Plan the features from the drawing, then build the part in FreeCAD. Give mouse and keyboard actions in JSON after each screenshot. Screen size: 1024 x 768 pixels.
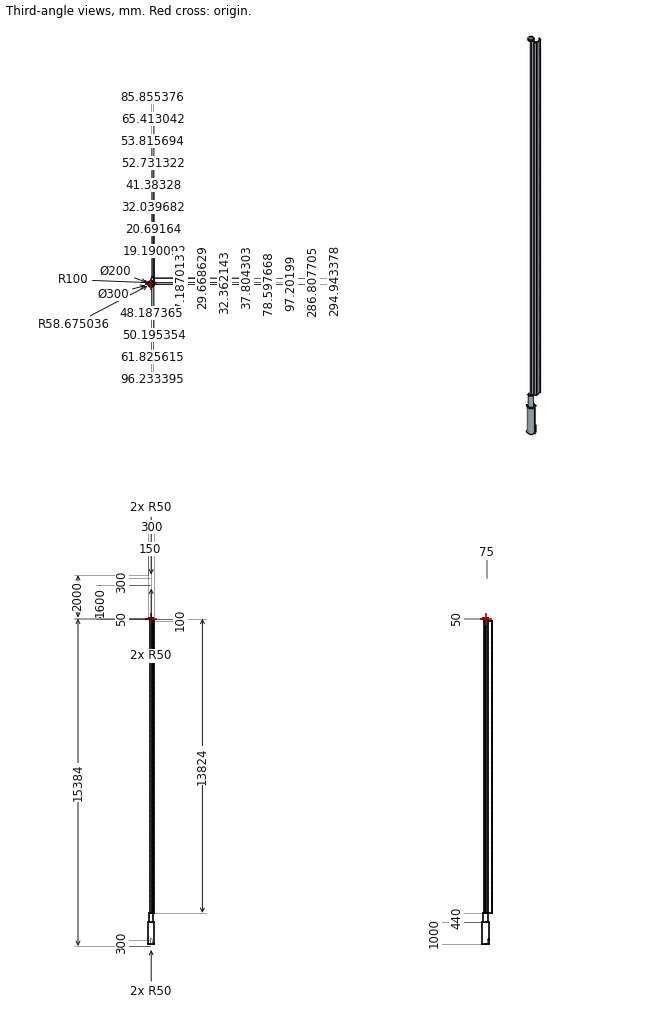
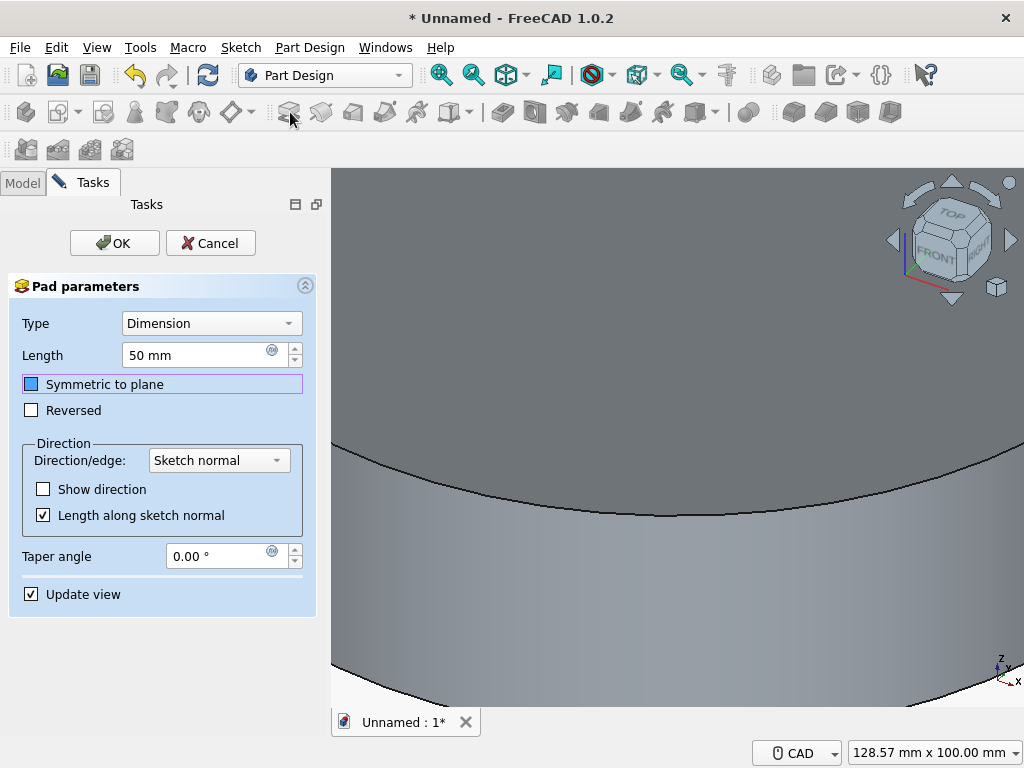
{"action": "left_click", "coordinate": [115, 243]}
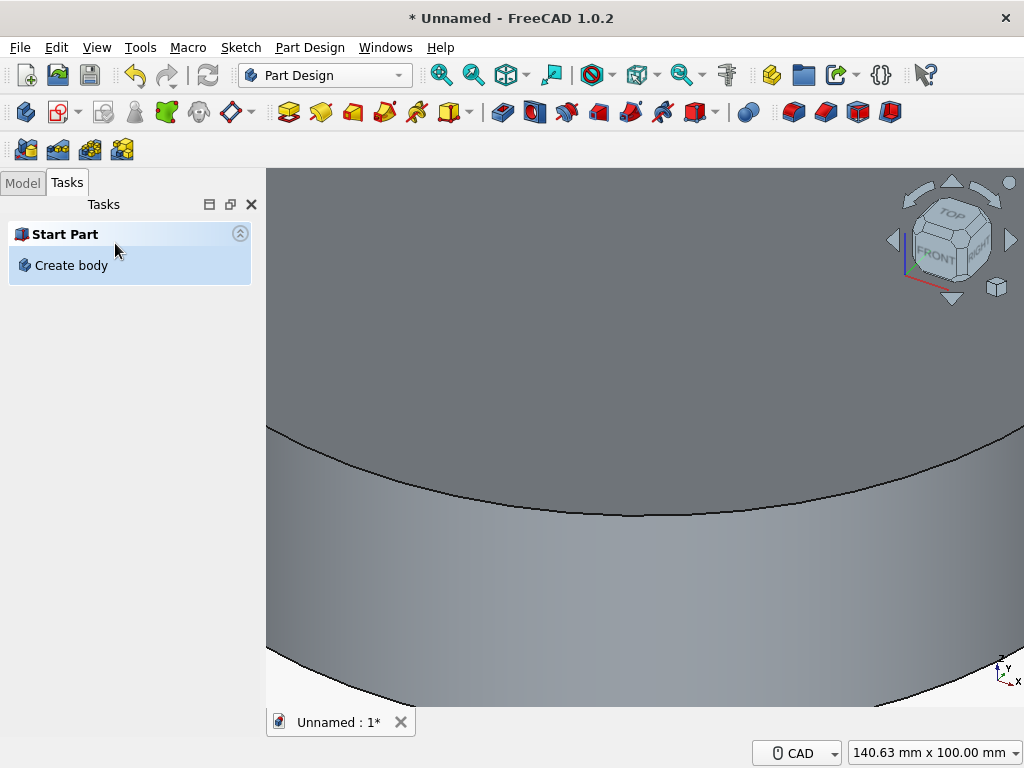
{"action": "left_click", "coordinate": [442, 76]}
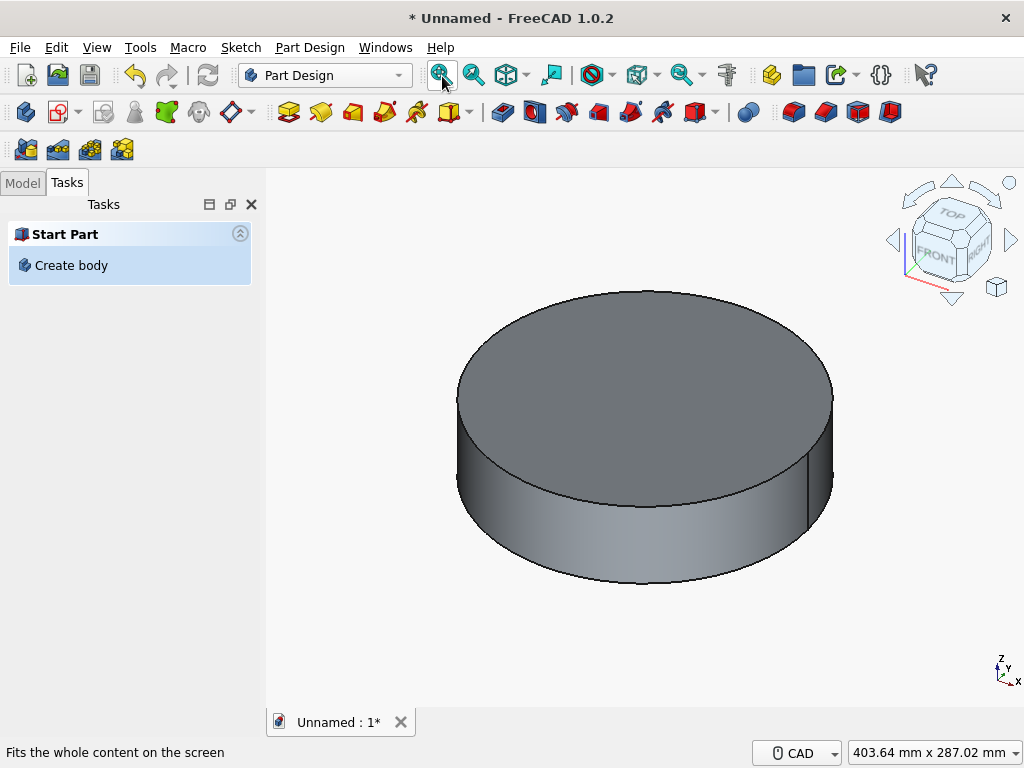
{"action": "left_click", "coordinate": [58, 112]}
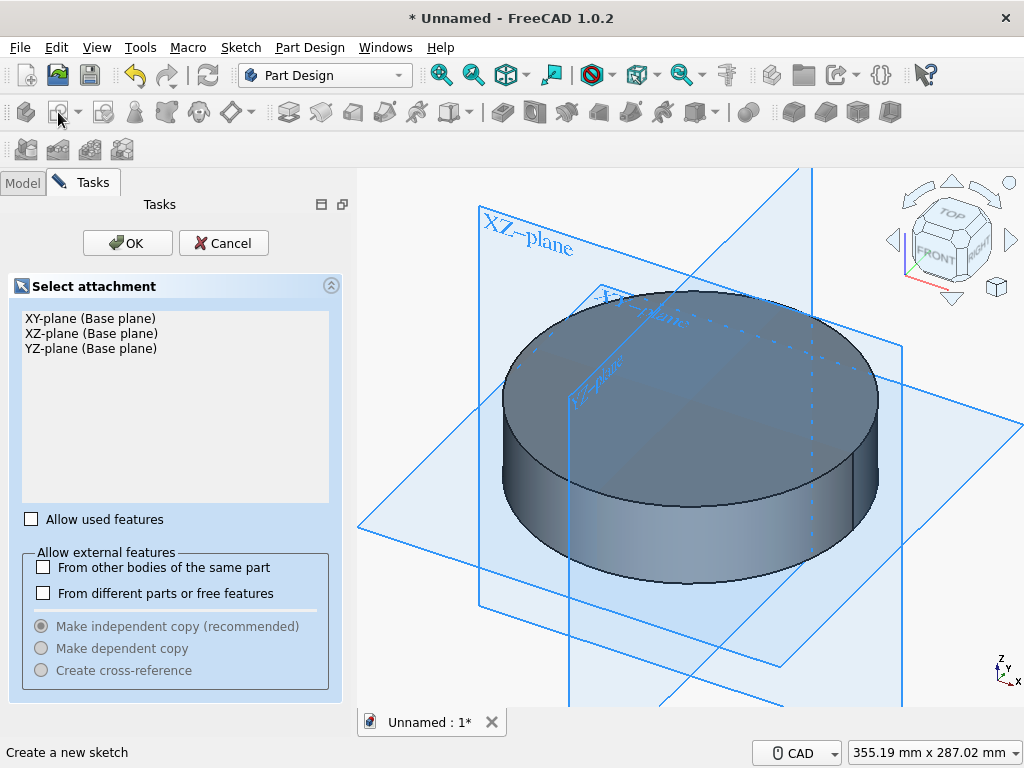
{"action": "left_click", "coordinate": [82, 318]}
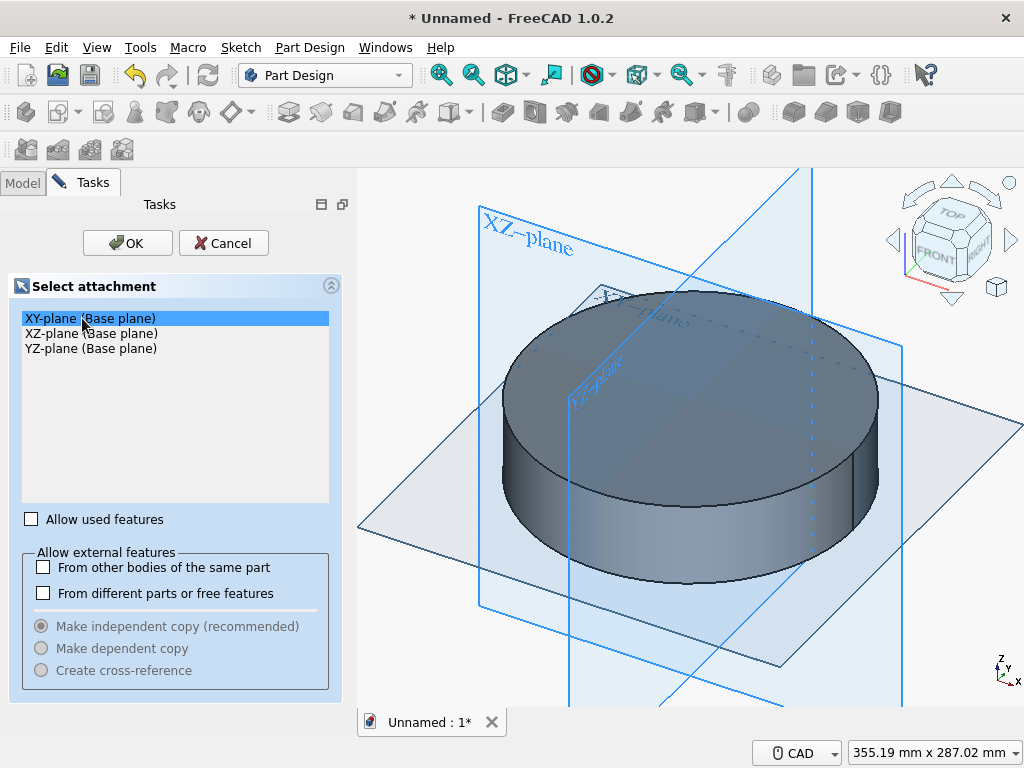
{"action": "left_click", "coordinate": [128, 243]}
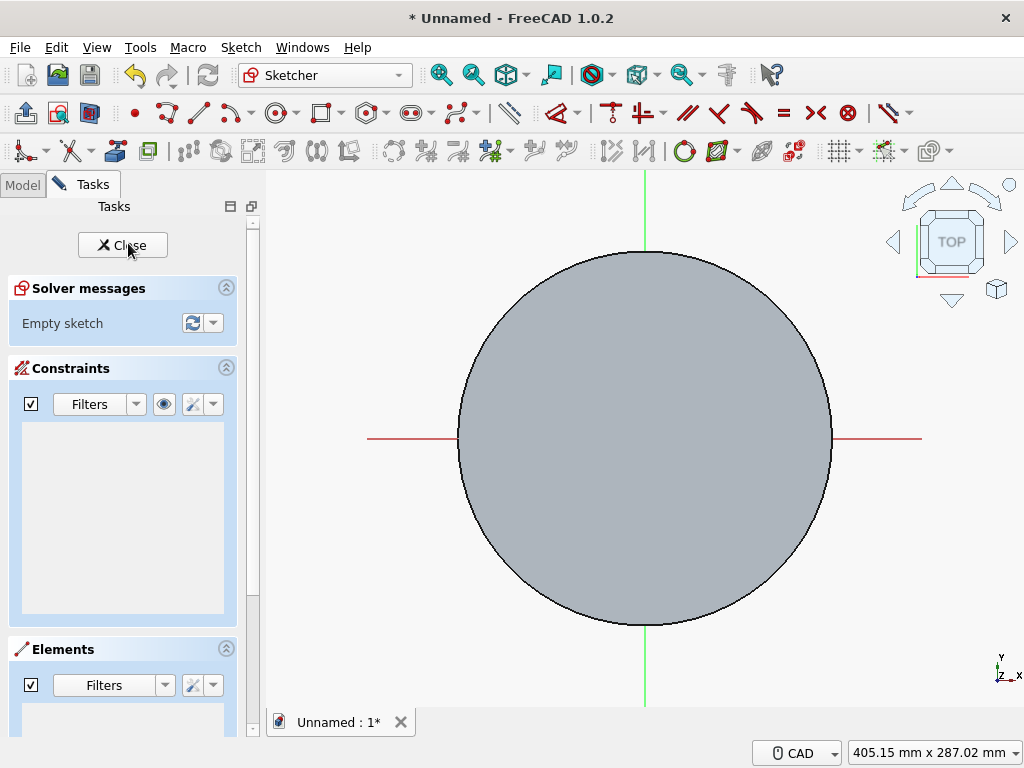
{"action": "left_click", "coordinate": [90, 114]}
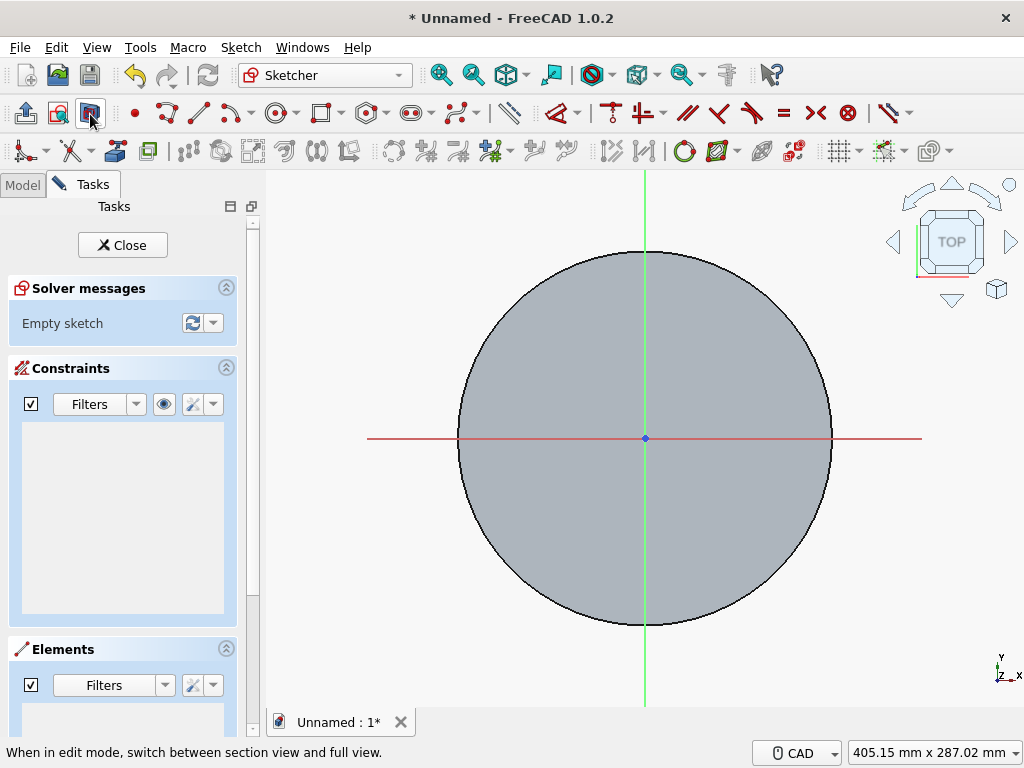
{"action": "scroll", "coordinate": [449, 661], "scroll_direction": "down", "scroll_amount": 4}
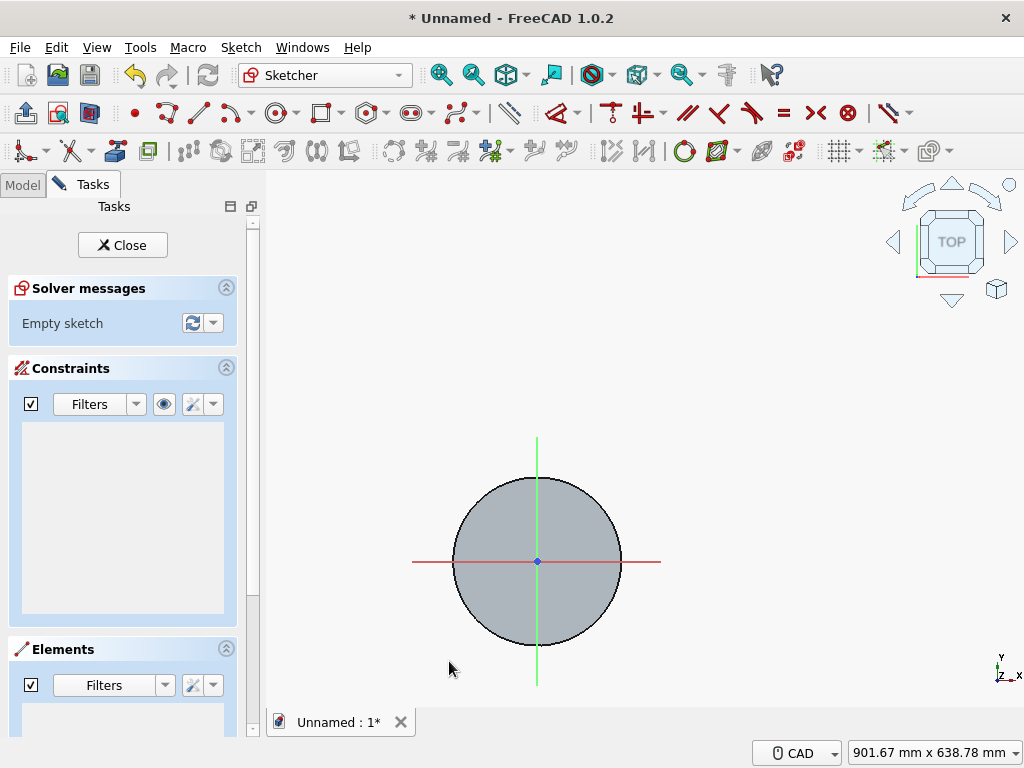
{"action": "left_click", "coordinate": [168, 114]}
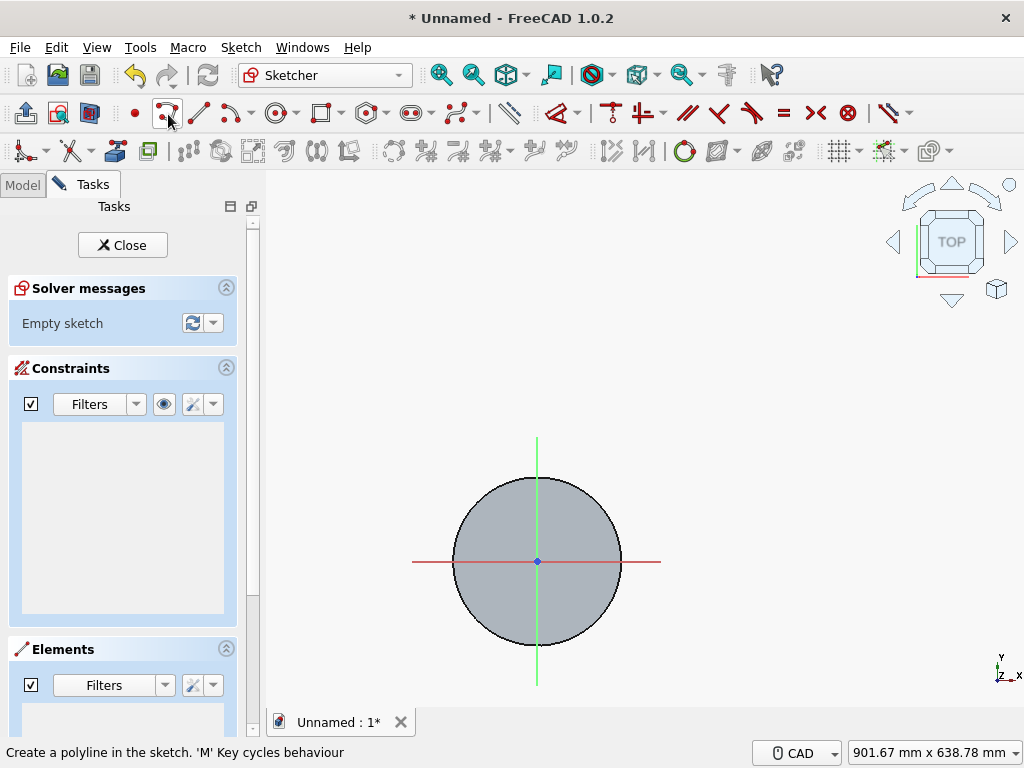
{"action": "left_click", "coordinate": [537, 512]}
{"action": "left_click", "coordinate": [589, 495]}
{"action": "left_click", "coordinate": [644, 468]}
{"action": "left_click", "coordinate": [627, 320]}
{"action": "left_click", "coordinate": [582, 289]}
{"action": "left_click", "coordinate": [609, 289]}
{"action": "left_click", "coordinate": [644, 314]}
{"action": "left_click", "coordinate": [660, 480]}
{"action": "left_click", "coordinate": [618, 539]}
{"action": "left_click", "coordinate": [578, 590]}
{"action": "right_click", "coordinate": [578, 590]}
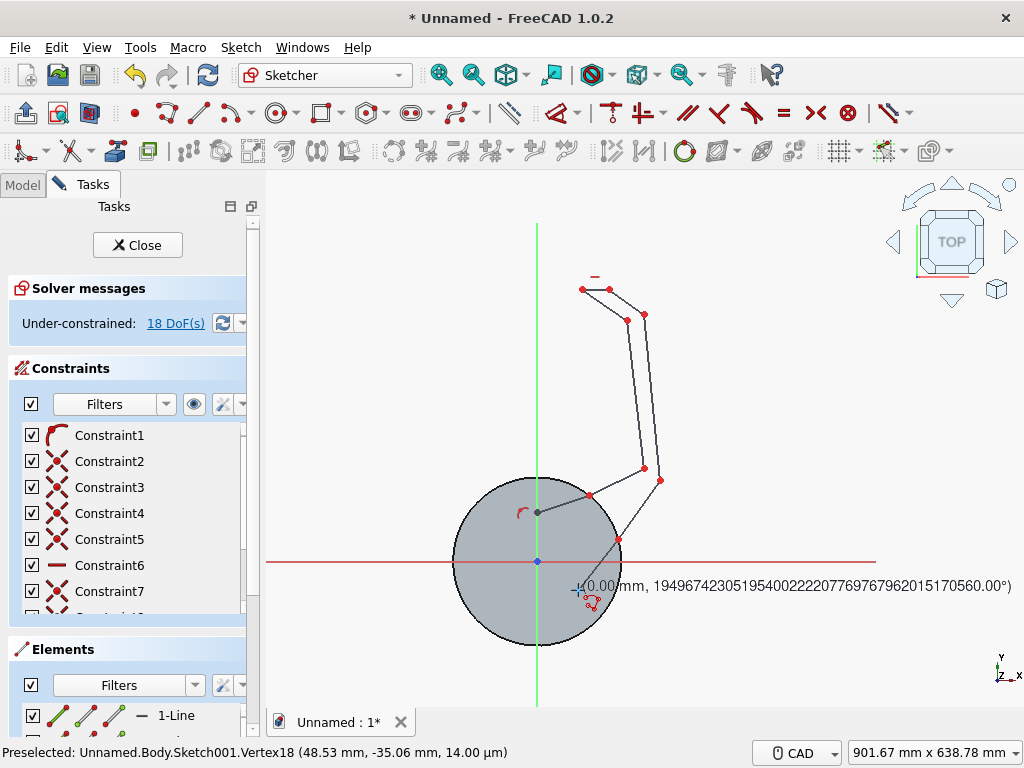
{"action": "left_click", "coordinate": [254, 114]}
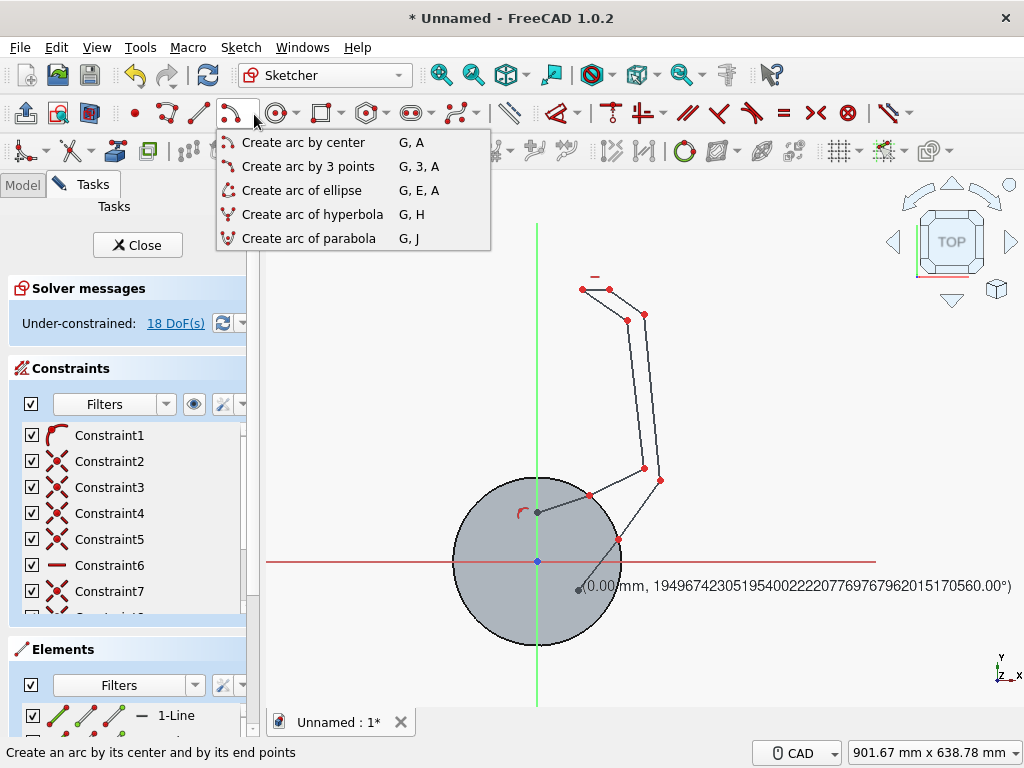
{"action": "left_click", "coordinate": [354, 166]}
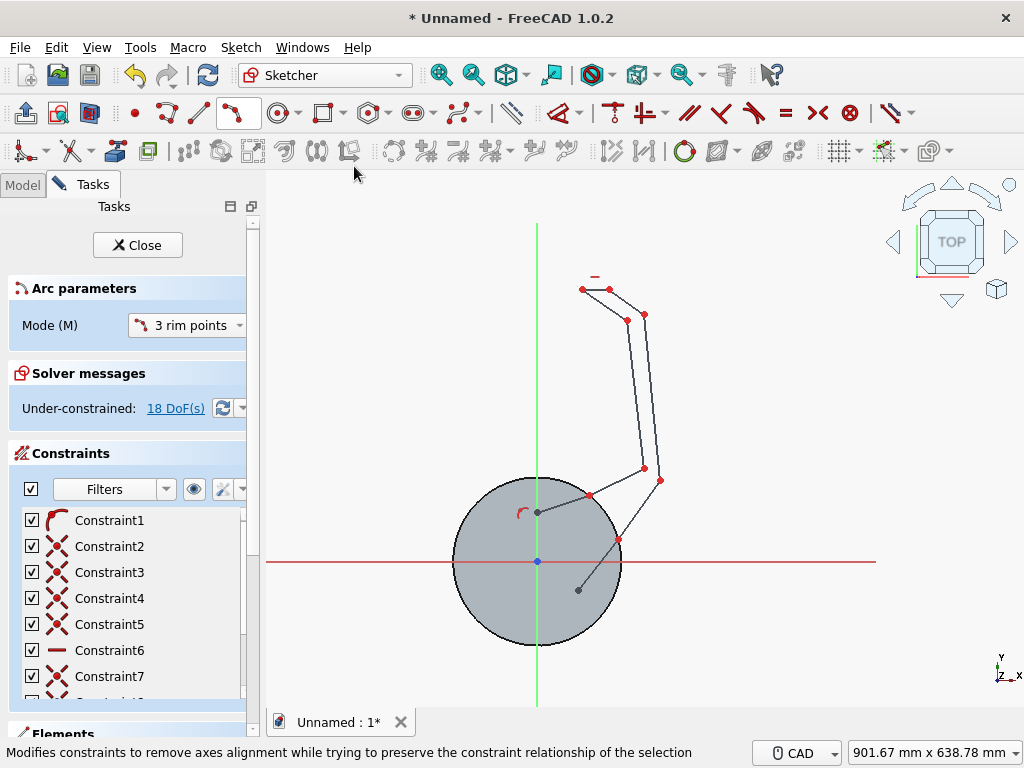
{"action": "left_click", "coordinate": [578, 591]}
{"action": "left_click", "coordinate": [537, 513]}
{"action": "left_click", "coordinate": [493, 584]}
{"action": "key", "text": "Escape"}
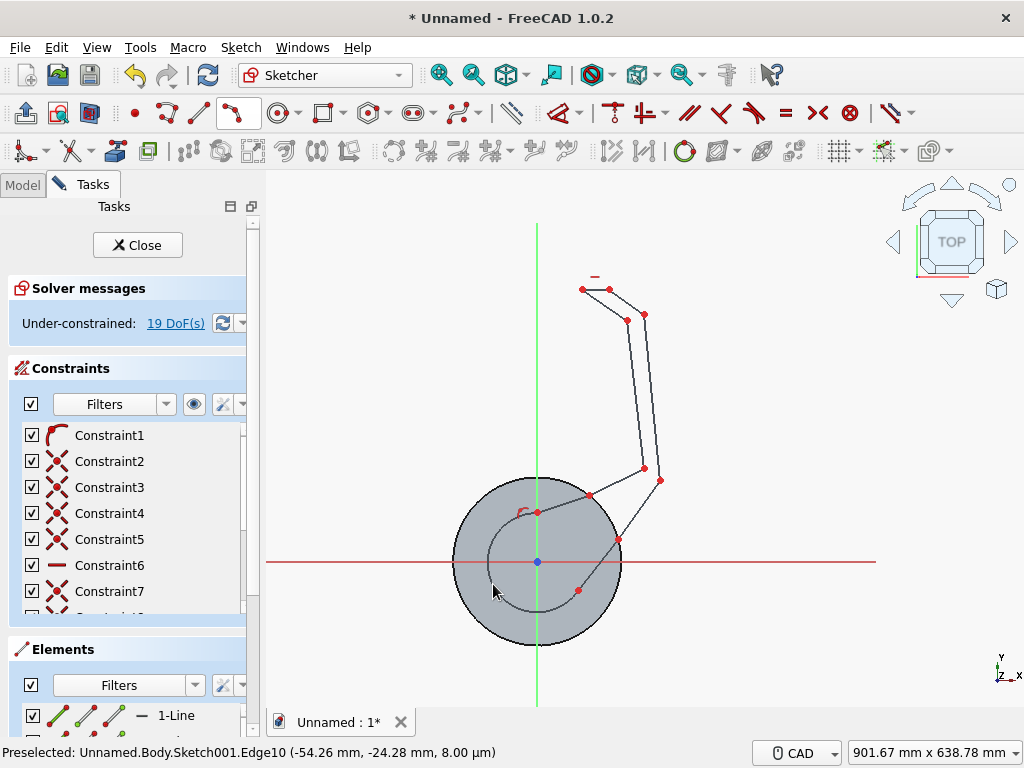
{"action": "left_click_drag", "start_coordinate": [527, 552], "coordinate": [547, 573]}